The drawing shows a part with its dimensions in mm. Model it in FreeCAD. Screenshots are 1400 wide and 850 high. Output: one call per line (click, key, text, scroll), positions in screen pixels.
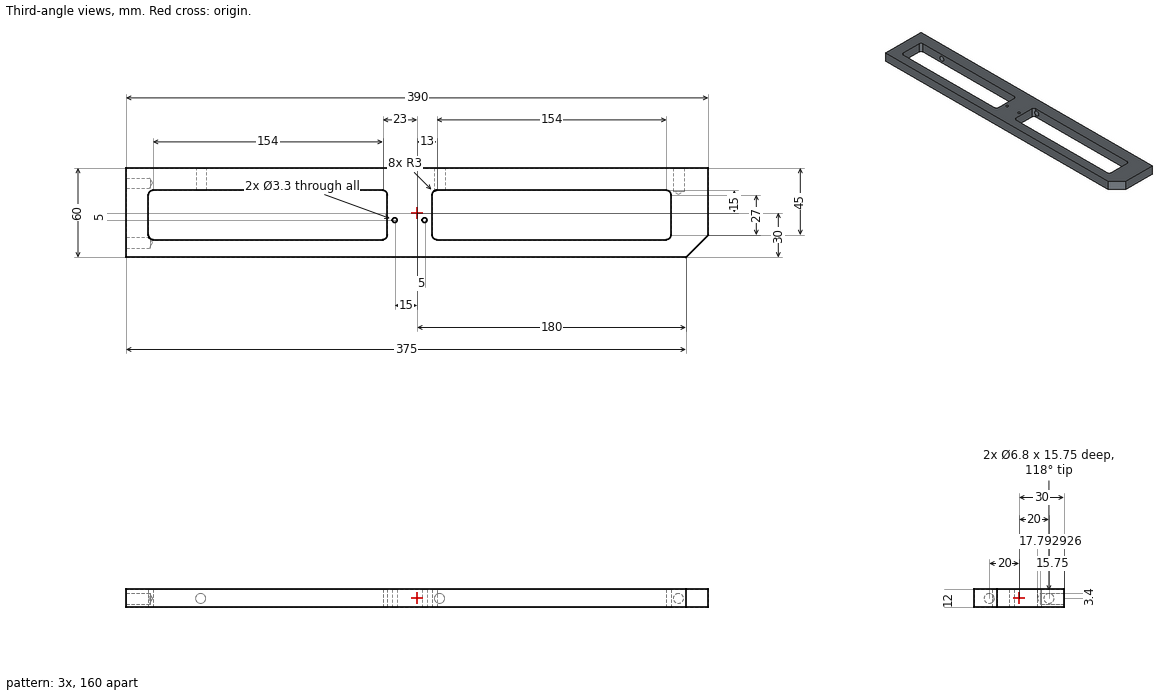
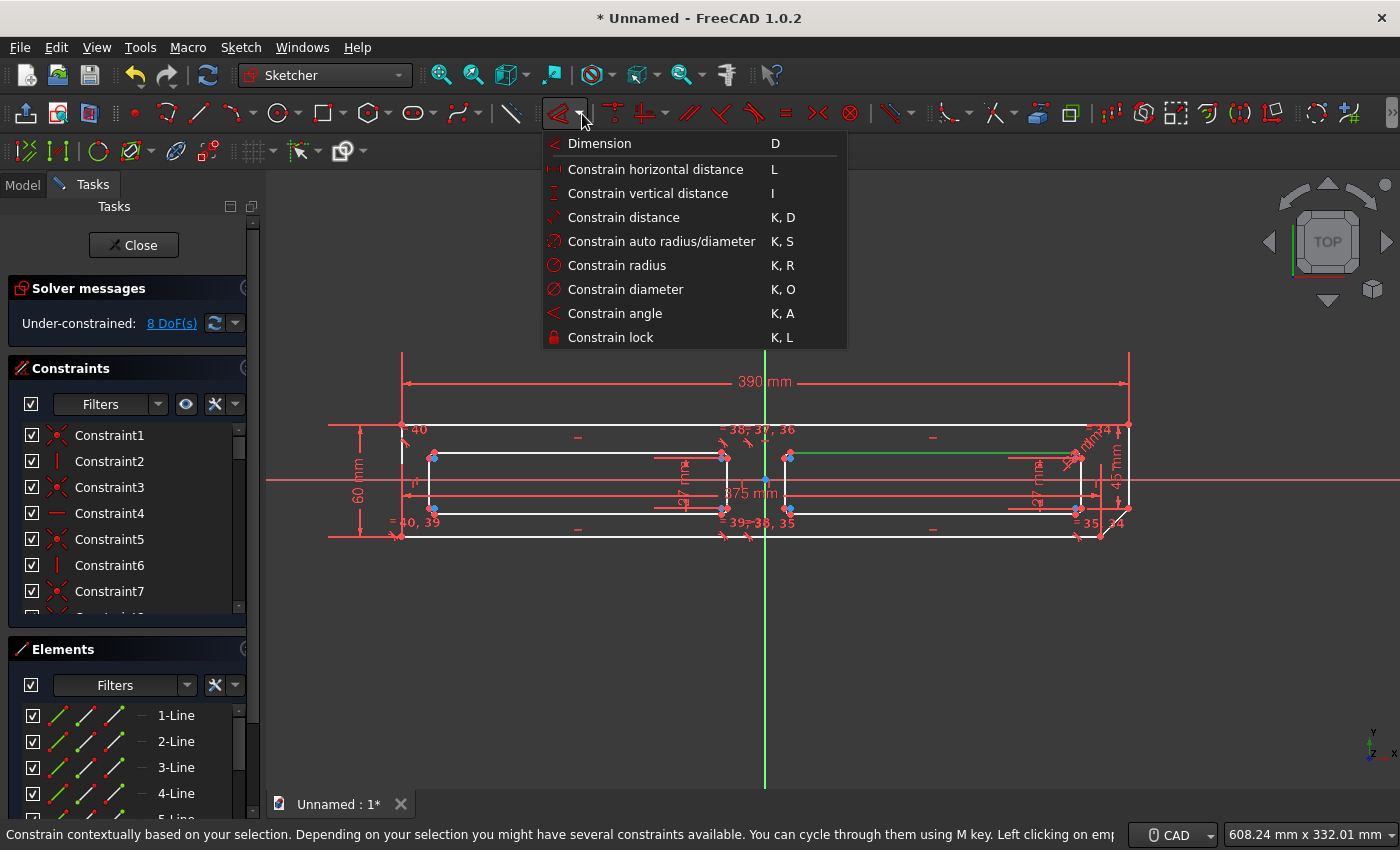
click(695, 169)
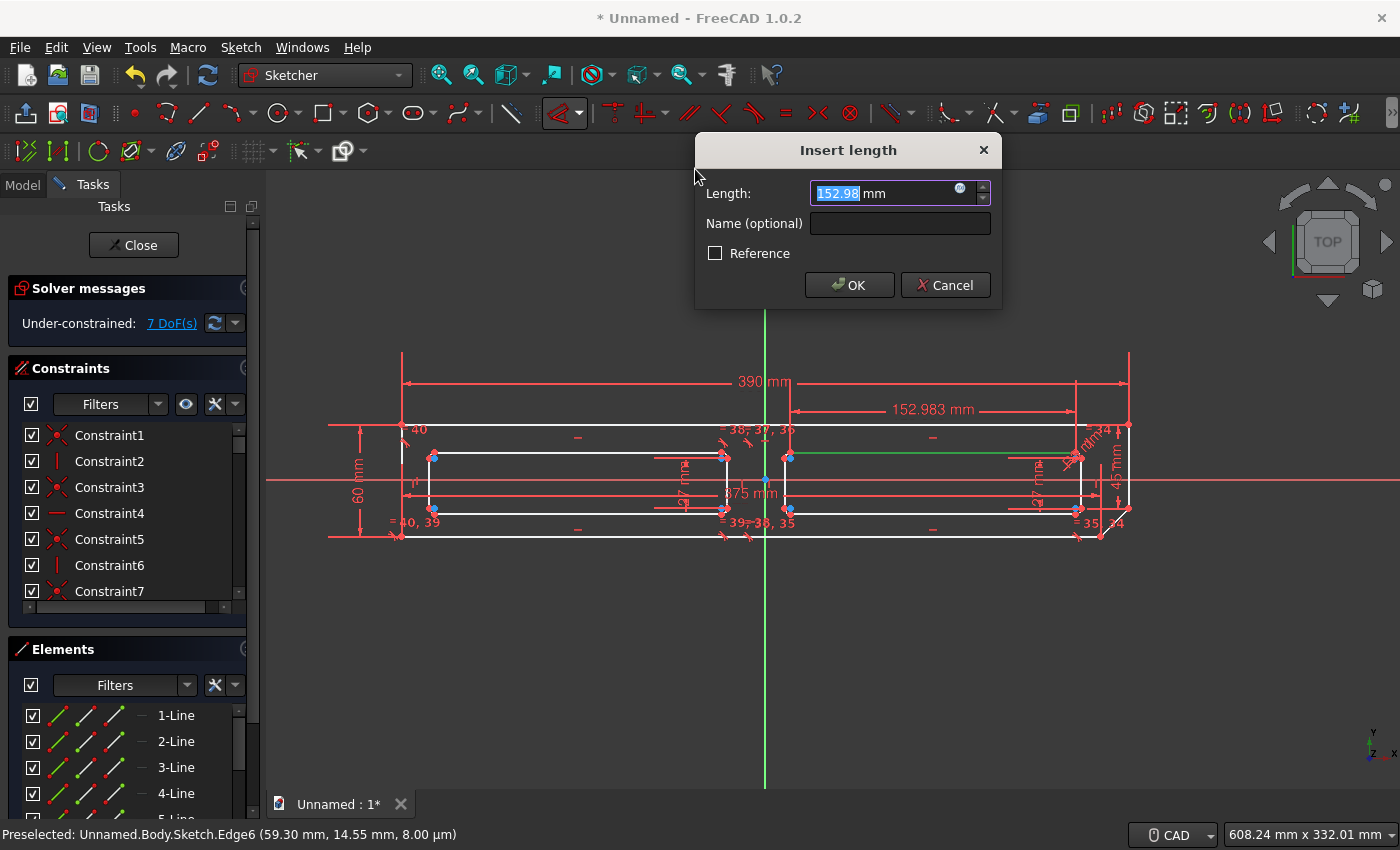
text(154)
key(Return)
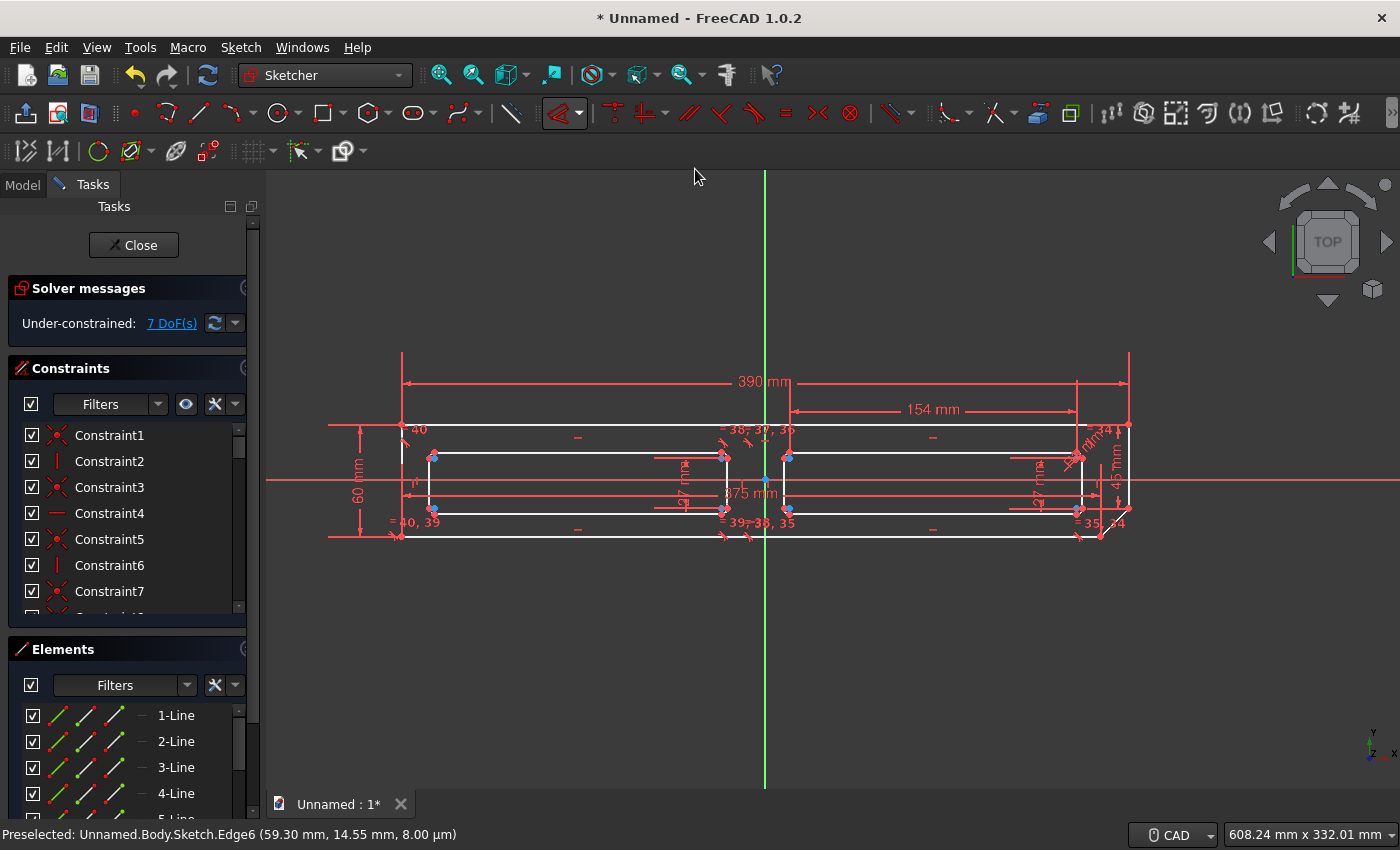
click(521, 453)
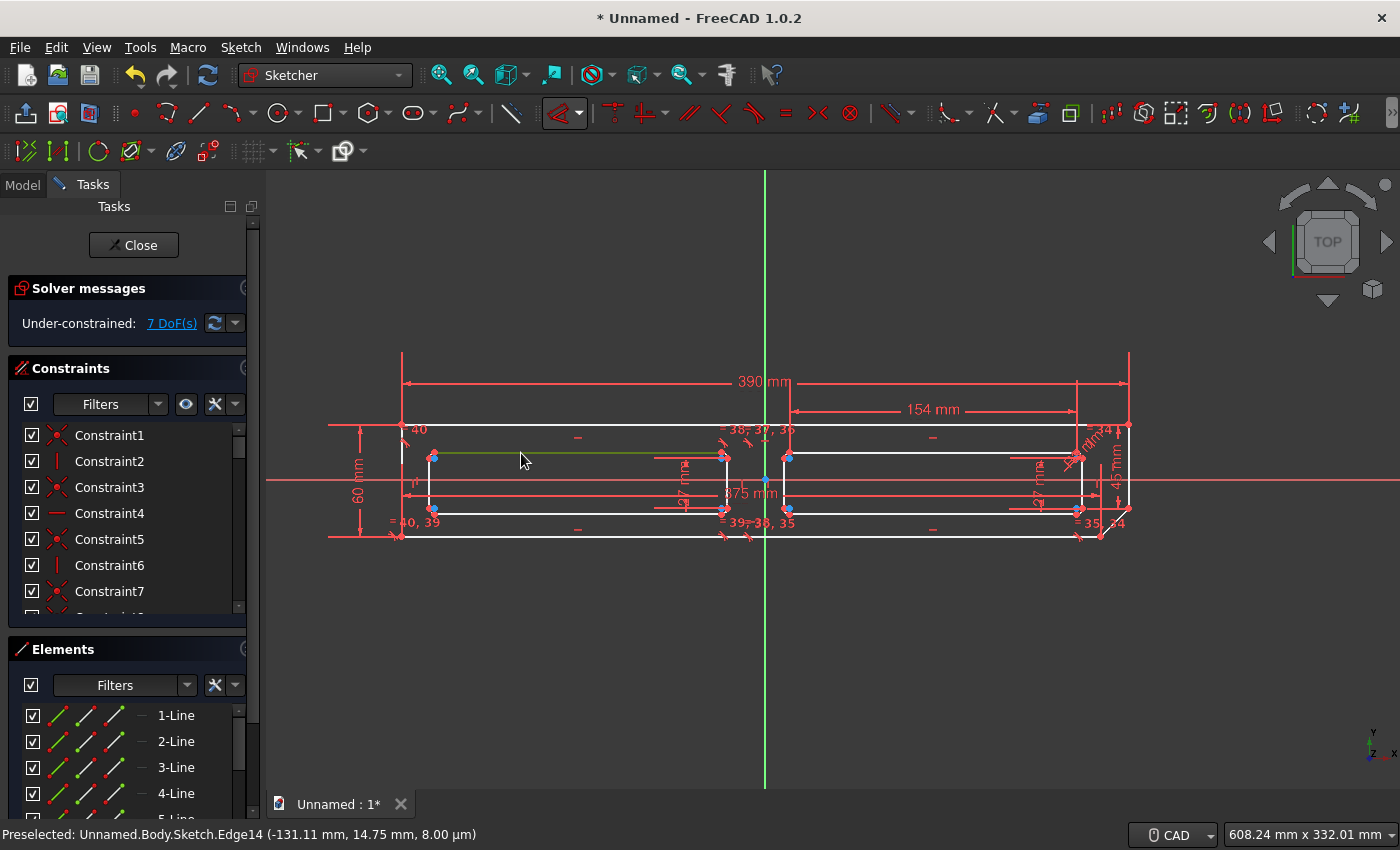
click(582, 114)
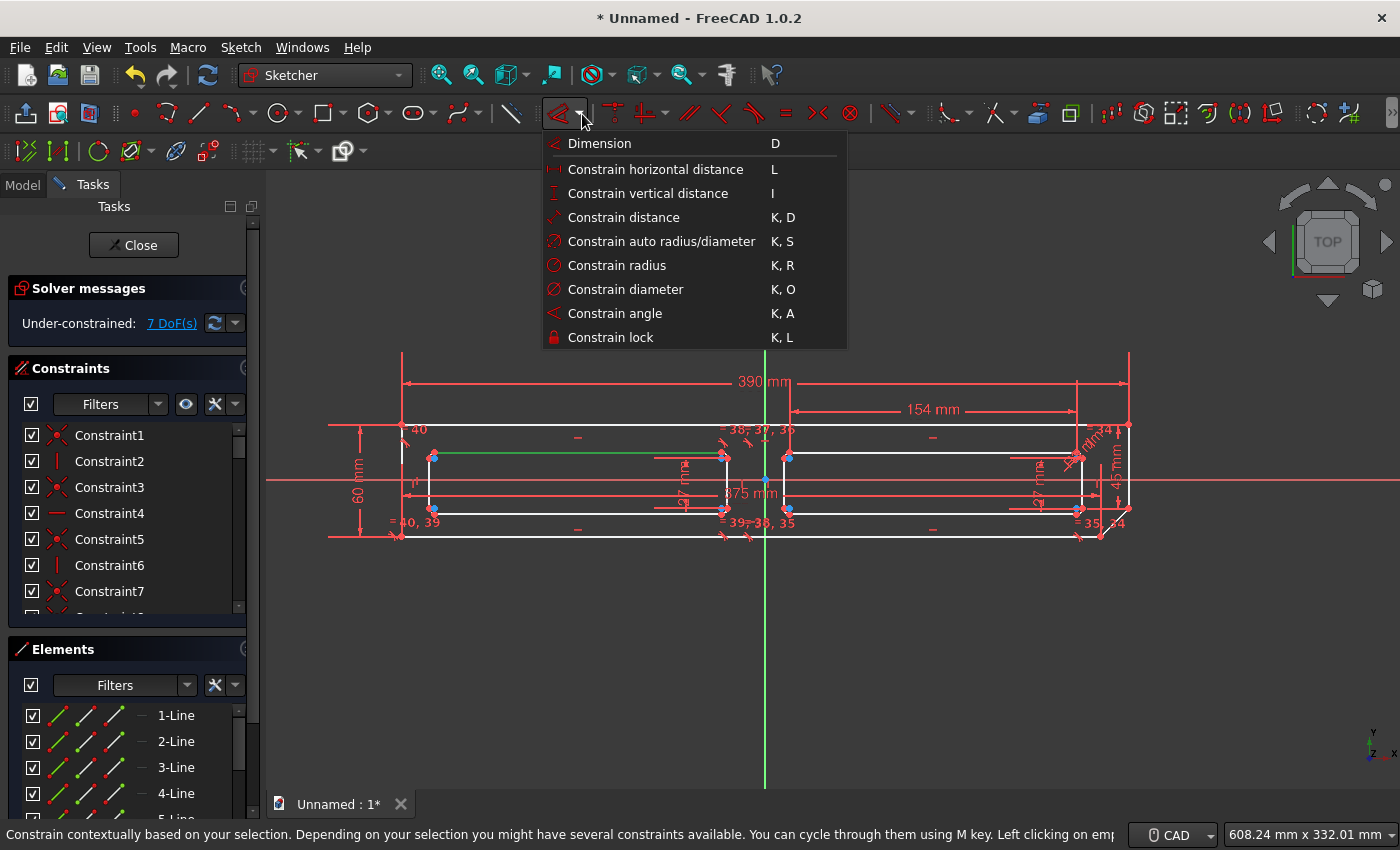
click(695, 169)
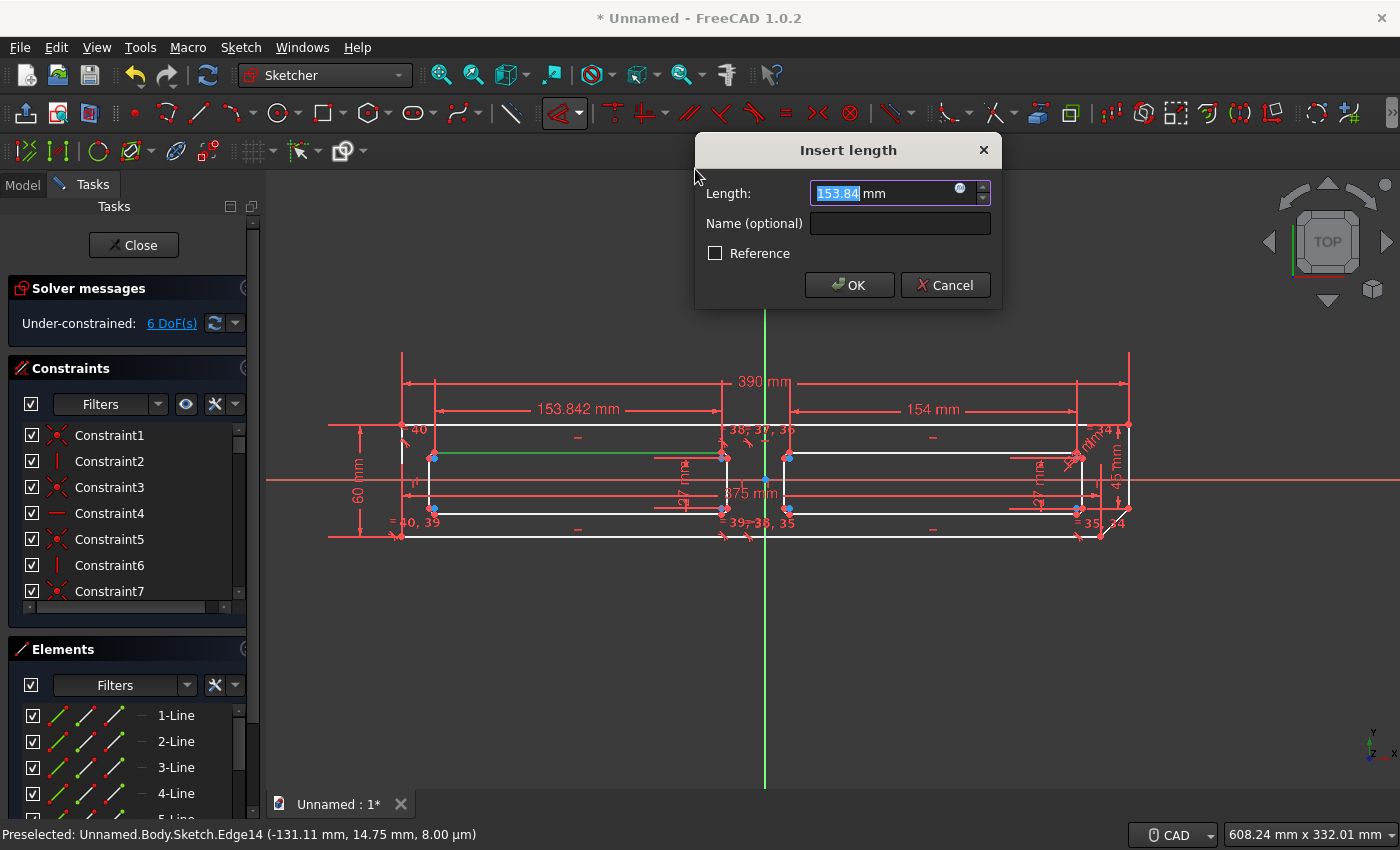
text(154)
key(Return)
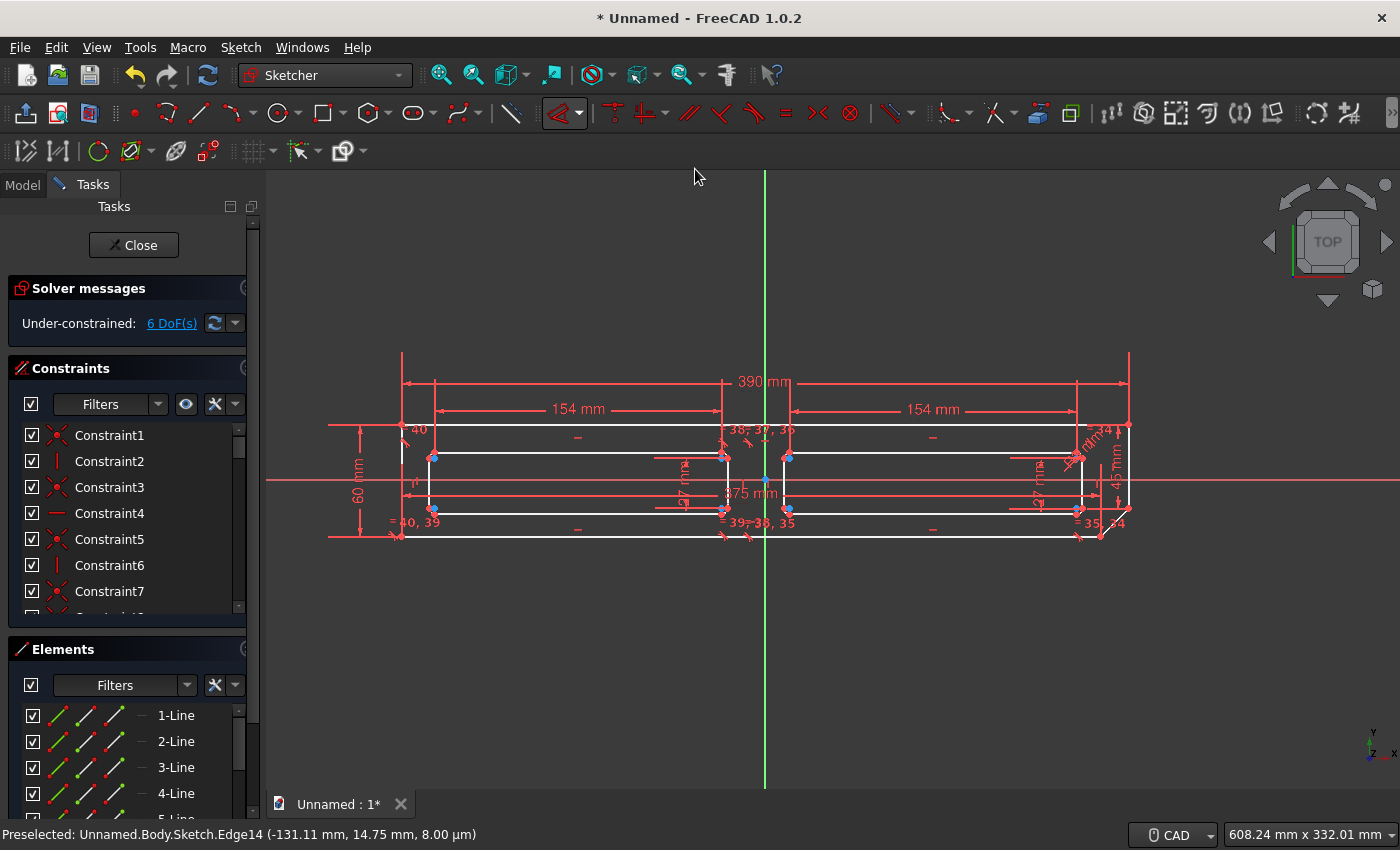
click(1101, 537)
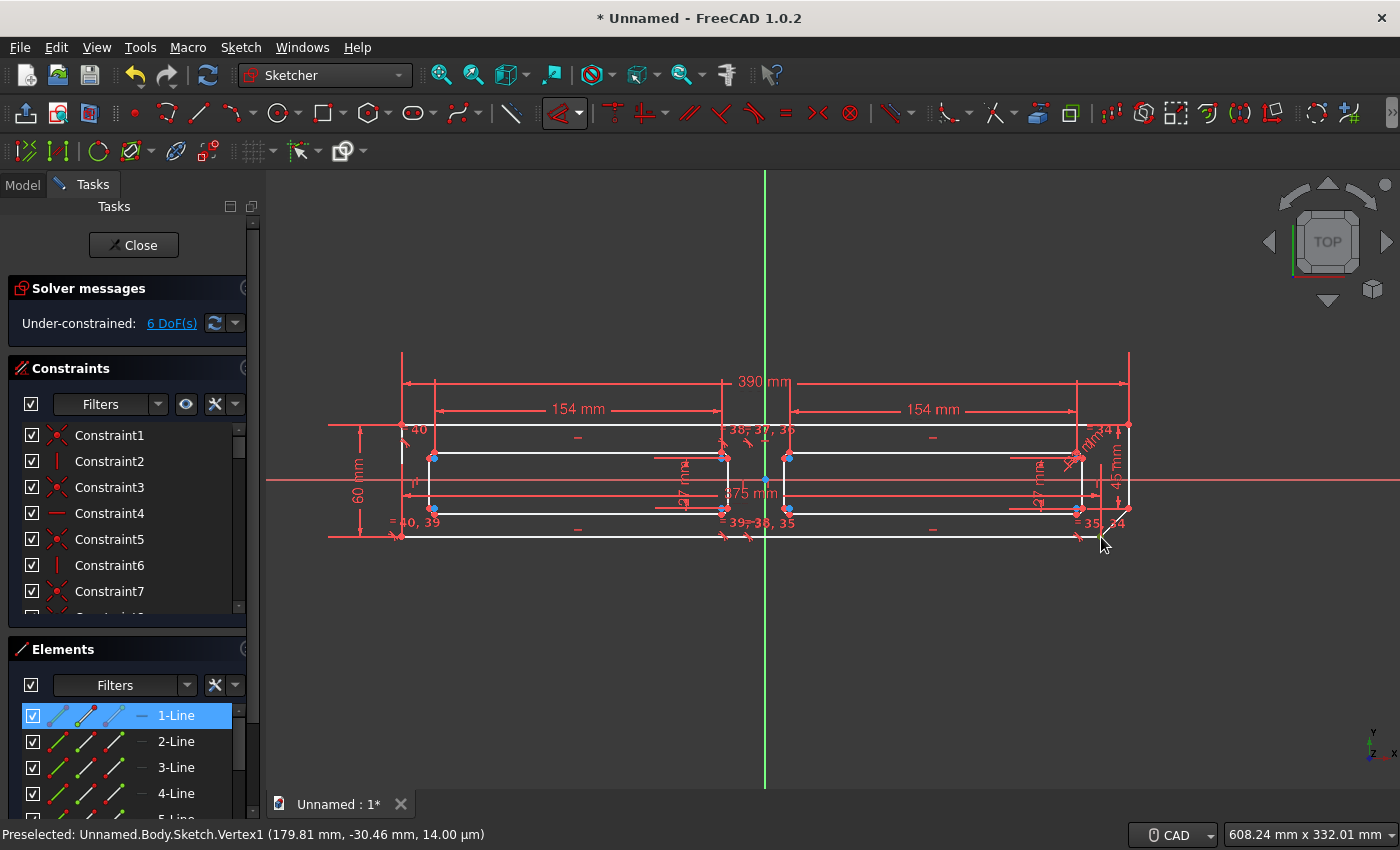
key(i)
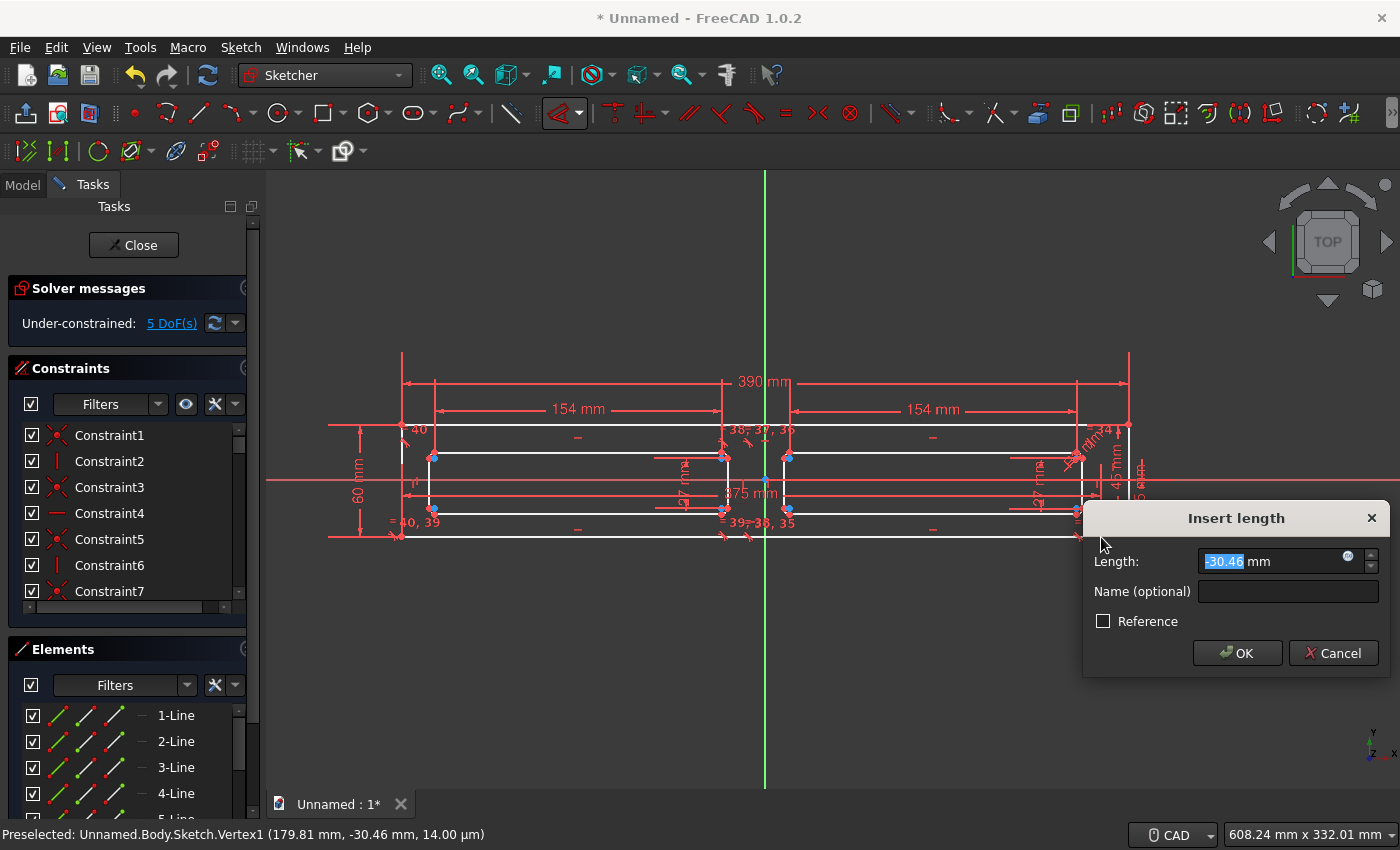
text(-30)
key(Return)